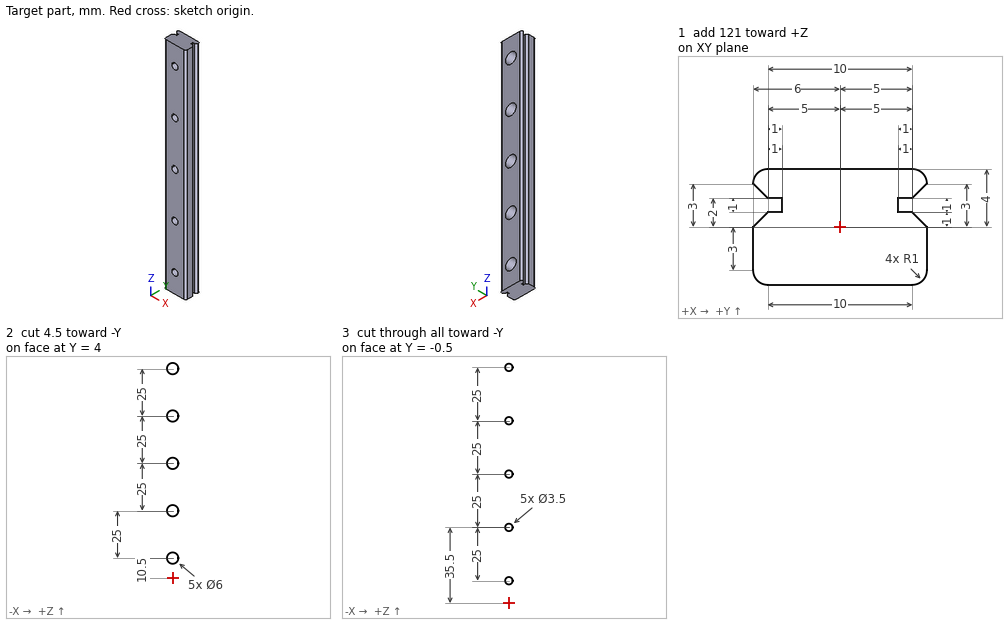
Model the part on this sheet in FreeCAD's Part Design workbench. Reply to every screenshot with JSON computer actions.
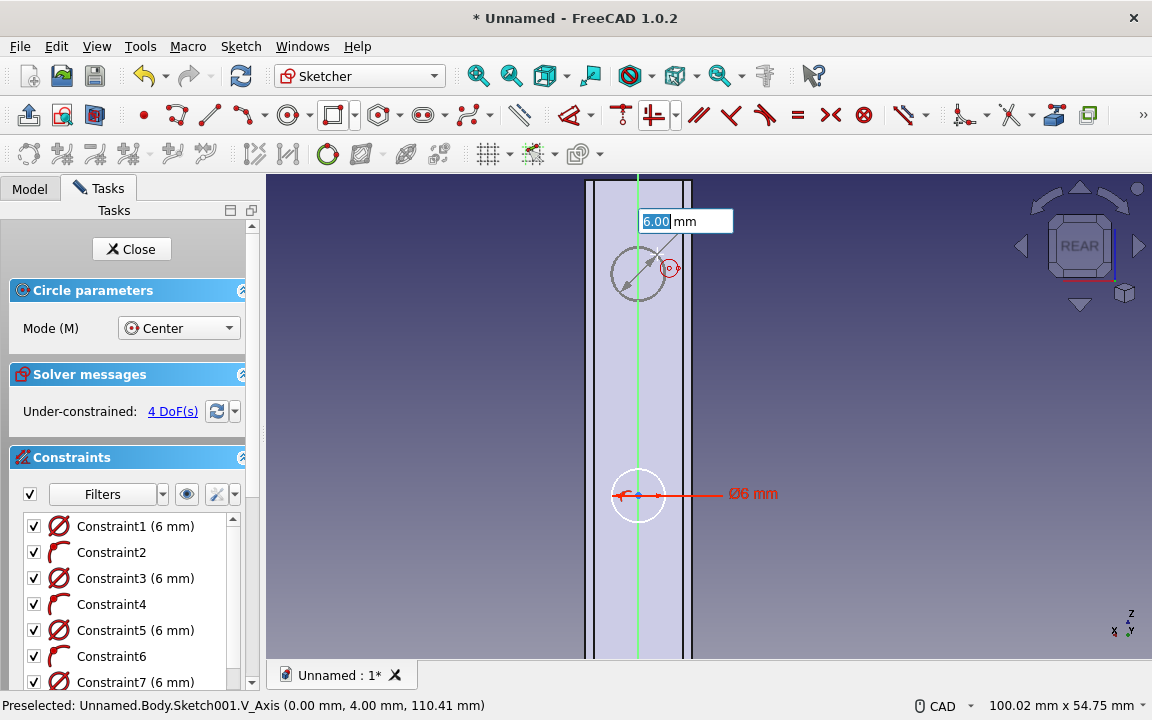
{"action": "type", "text": "6"}
{"action": "key", "text": "Return"}
{"action": "key", "text": "Escape"}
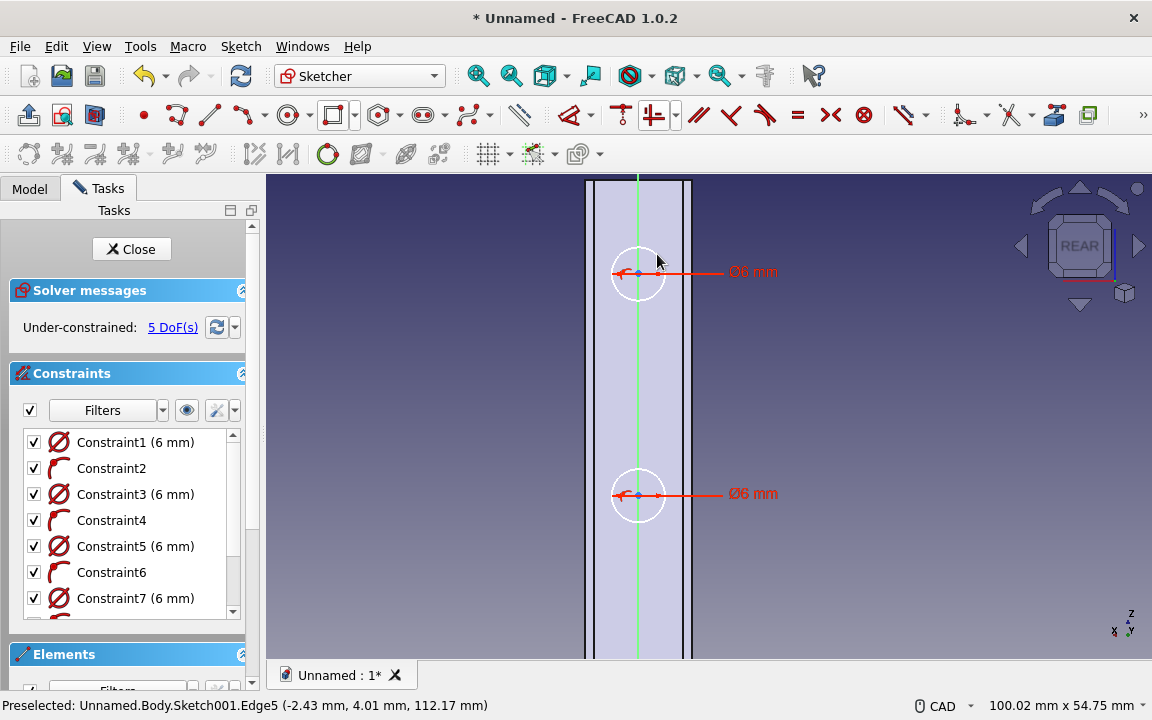
{"action": "left_click", "coordinate": [568, 116]}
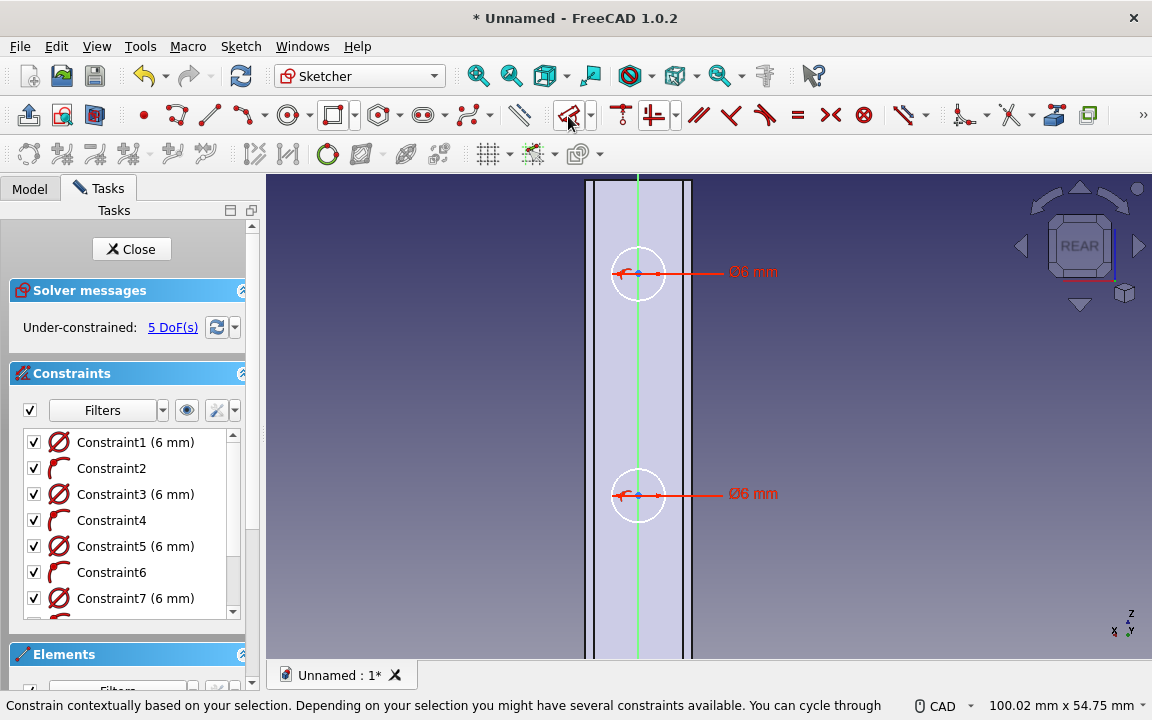
{"action": "scroll", "coordinate": [641, 273], "scroll_direction": "down", "scroll_amount": 6}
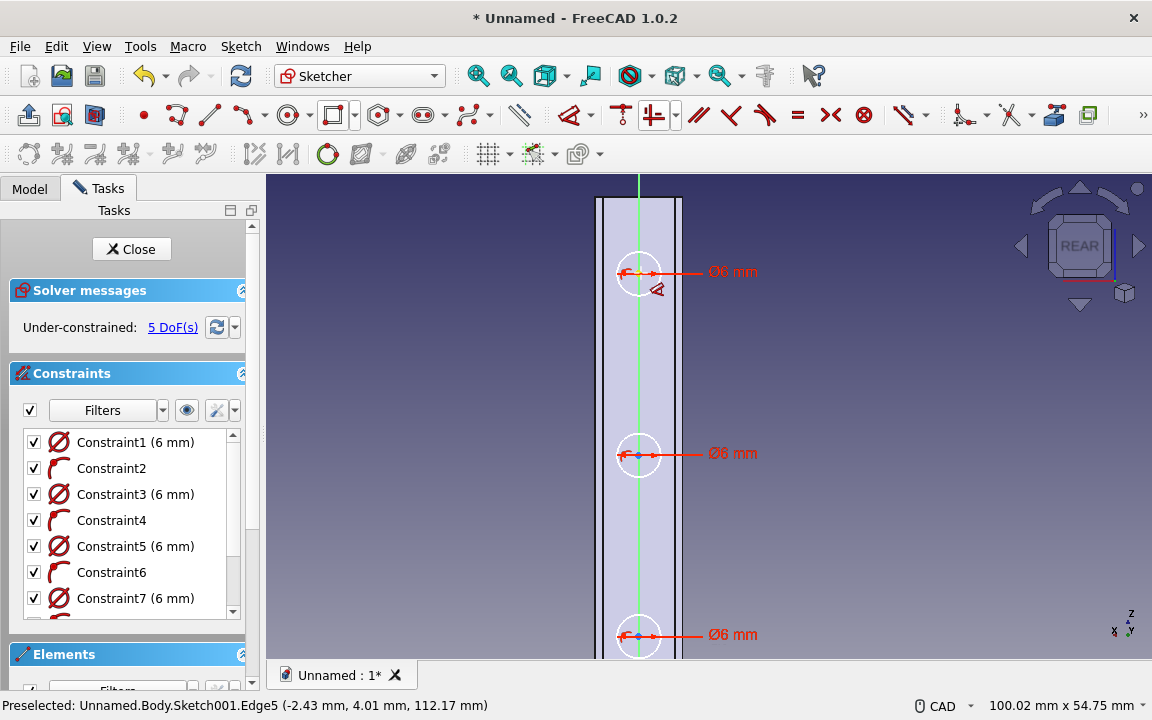
{"action": "left_click", "coordinate": [641, 540]}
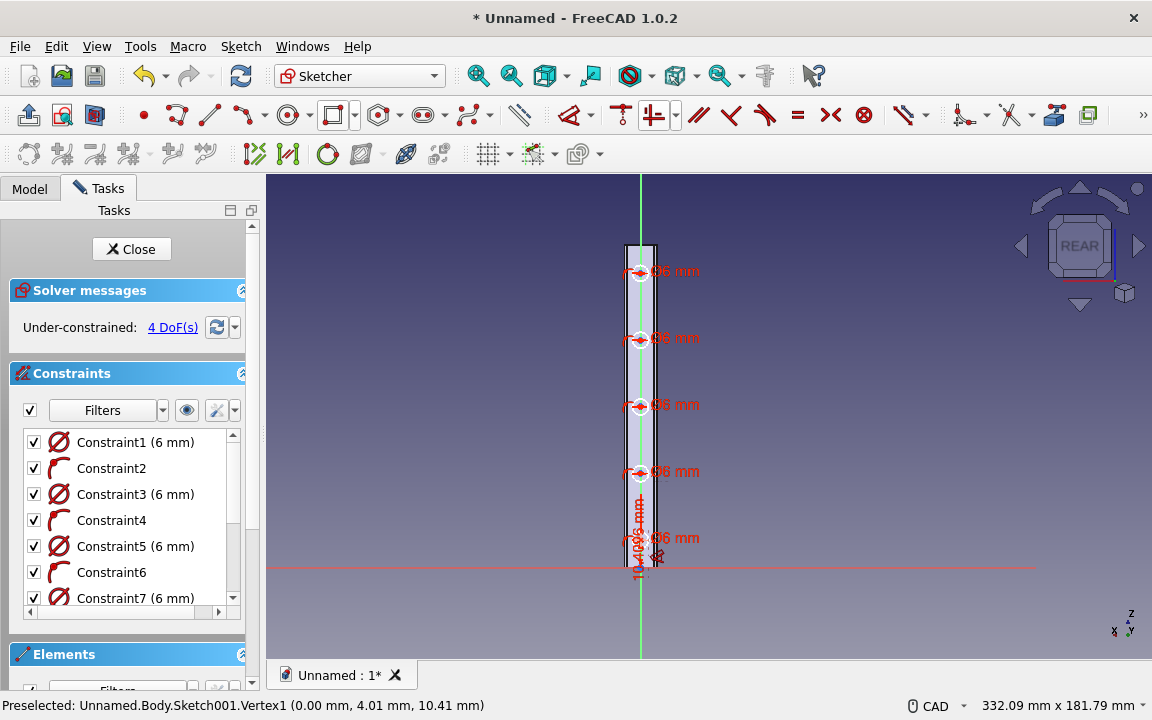
{"action": "left_click", "coordinate": [641, 474]}
{"action": "left_click", "coordinate": [675, 507]}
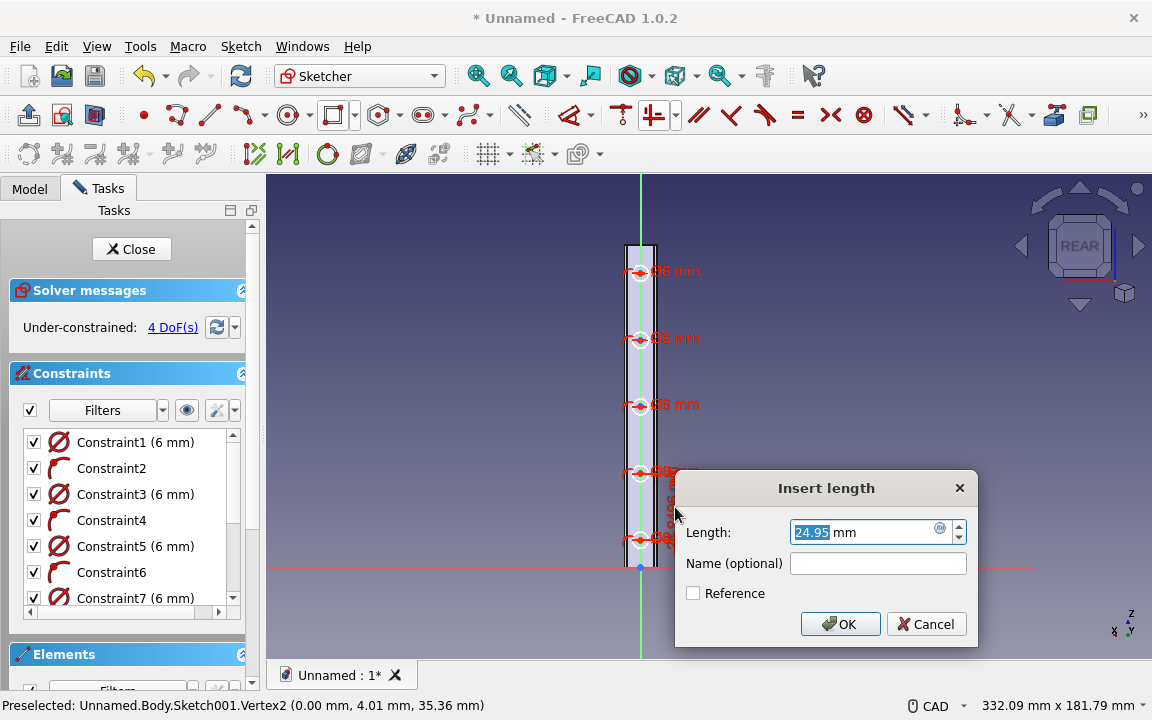
{"action": "type", "text": "25"}
{"action": "key", "text": "Return"}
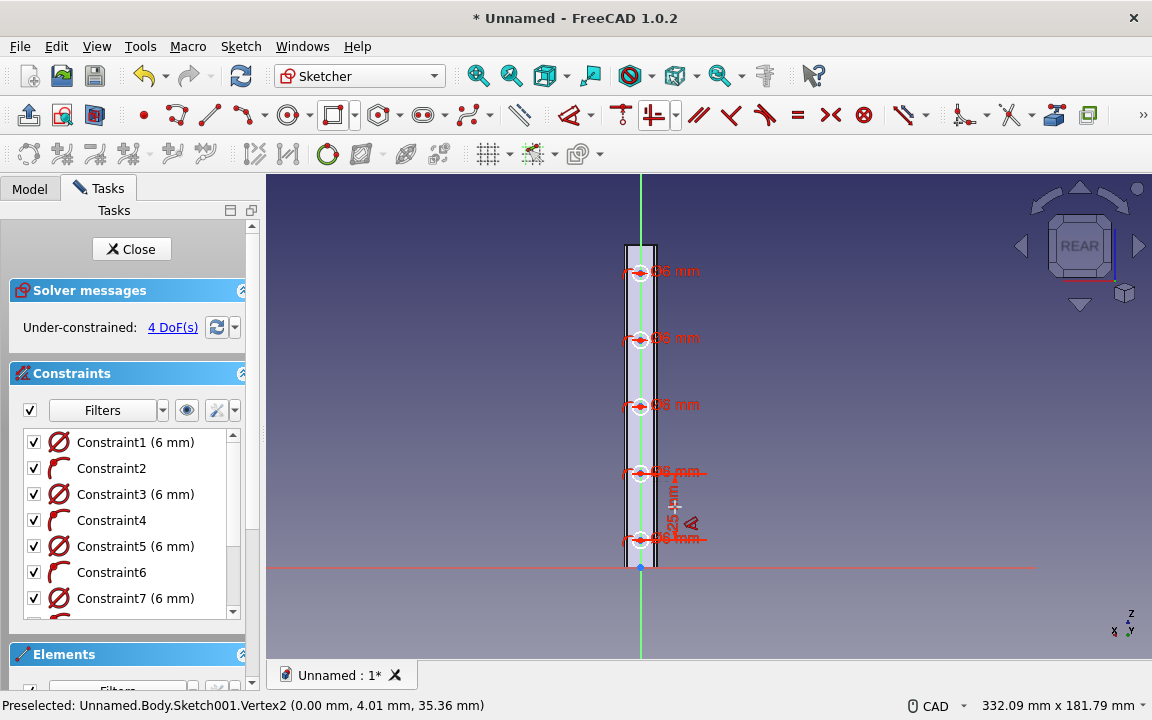
{"action": "left_click", "coordinate": [641, 474]}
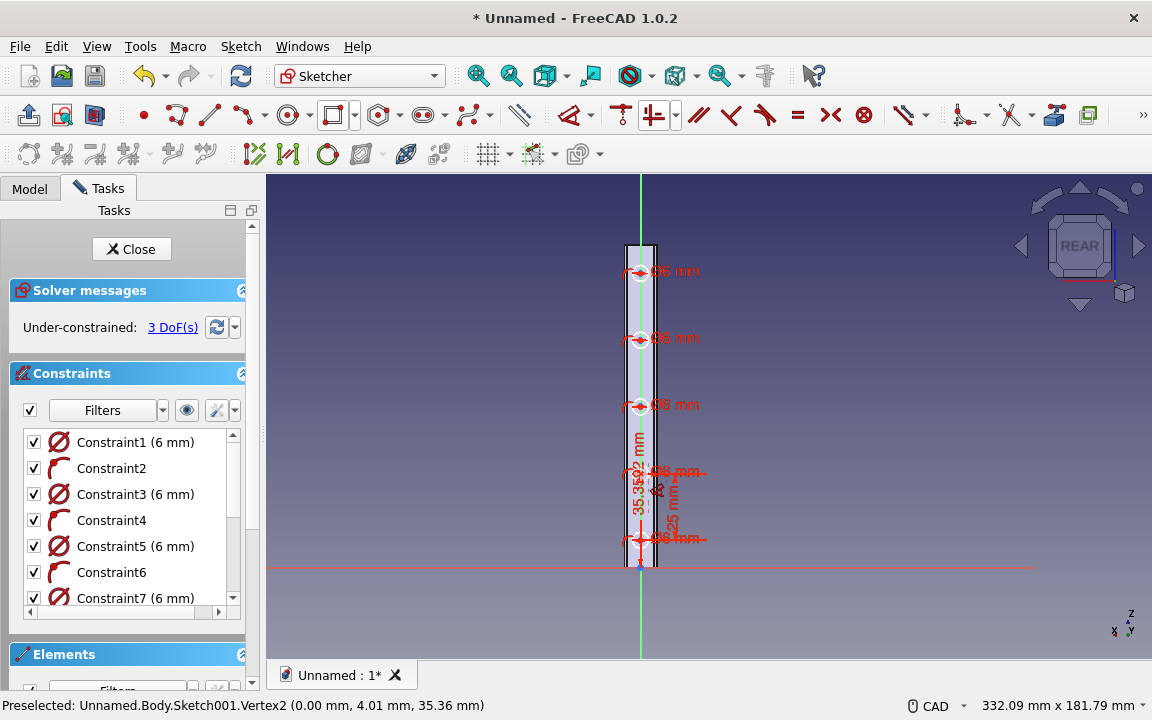
{"action": "left_click", "coordinate": [641, 407]}
{"action": "left_click", "coordinate": [675, 440]}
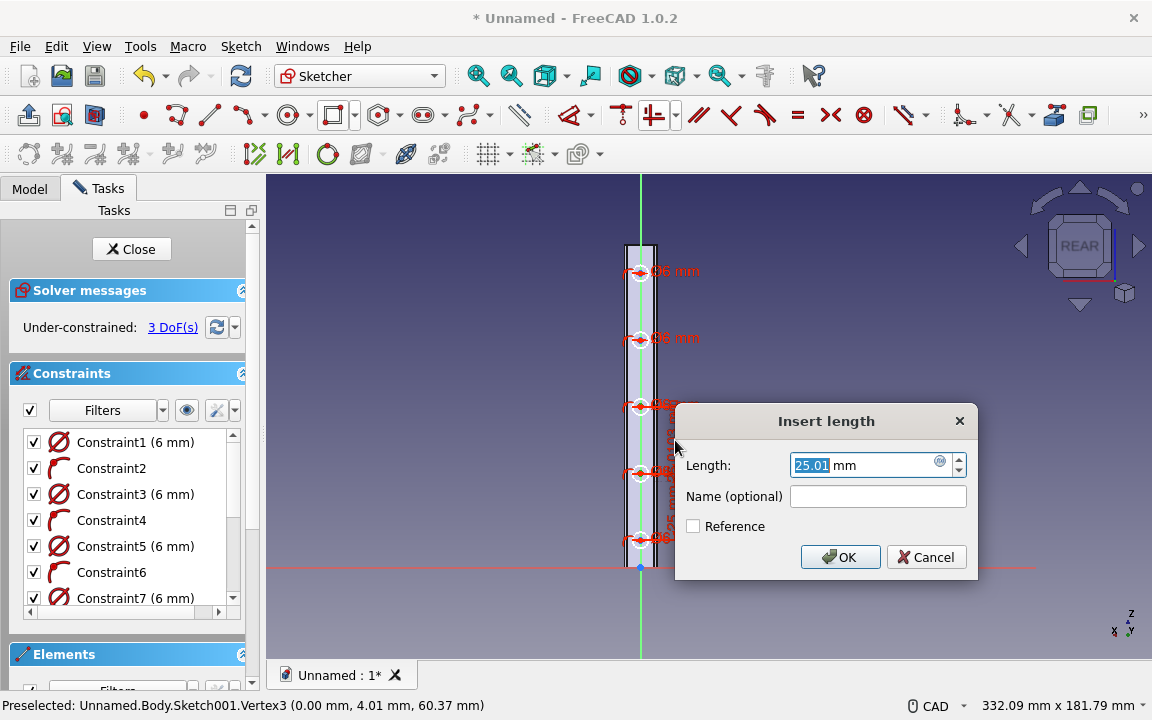
{"action": "type", "text": "25"}
{"action": "key", "text": "Return"}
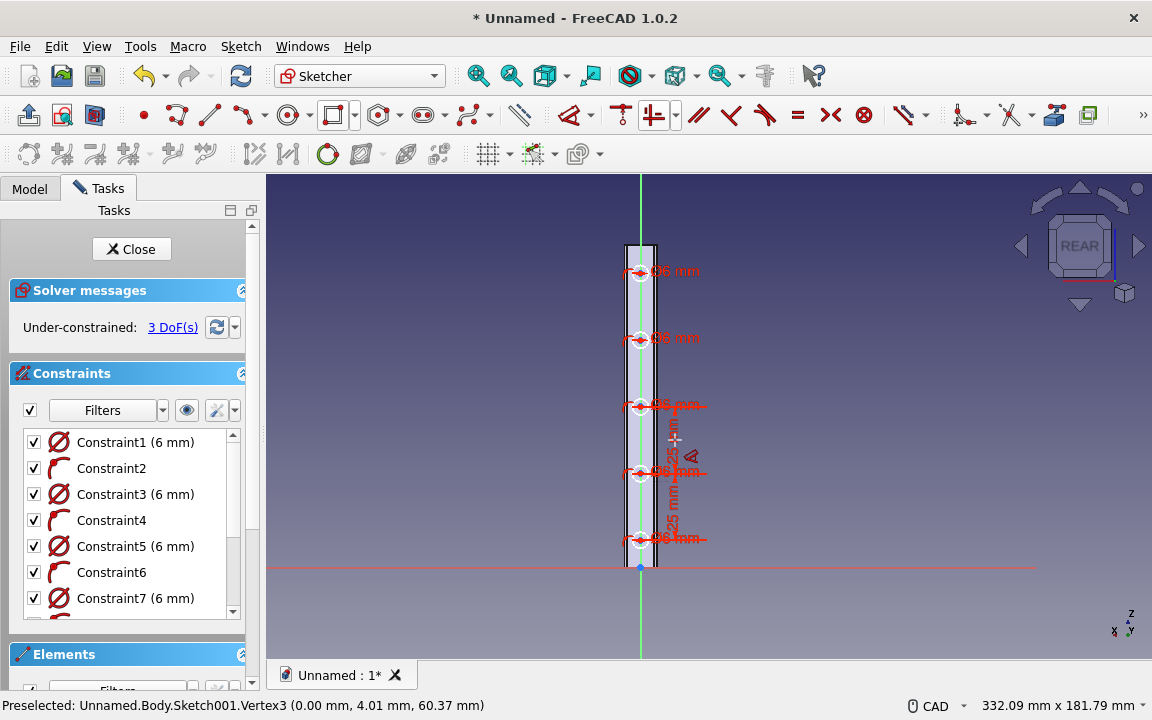
{"action": "left_click", "coordinate": [641, 407]}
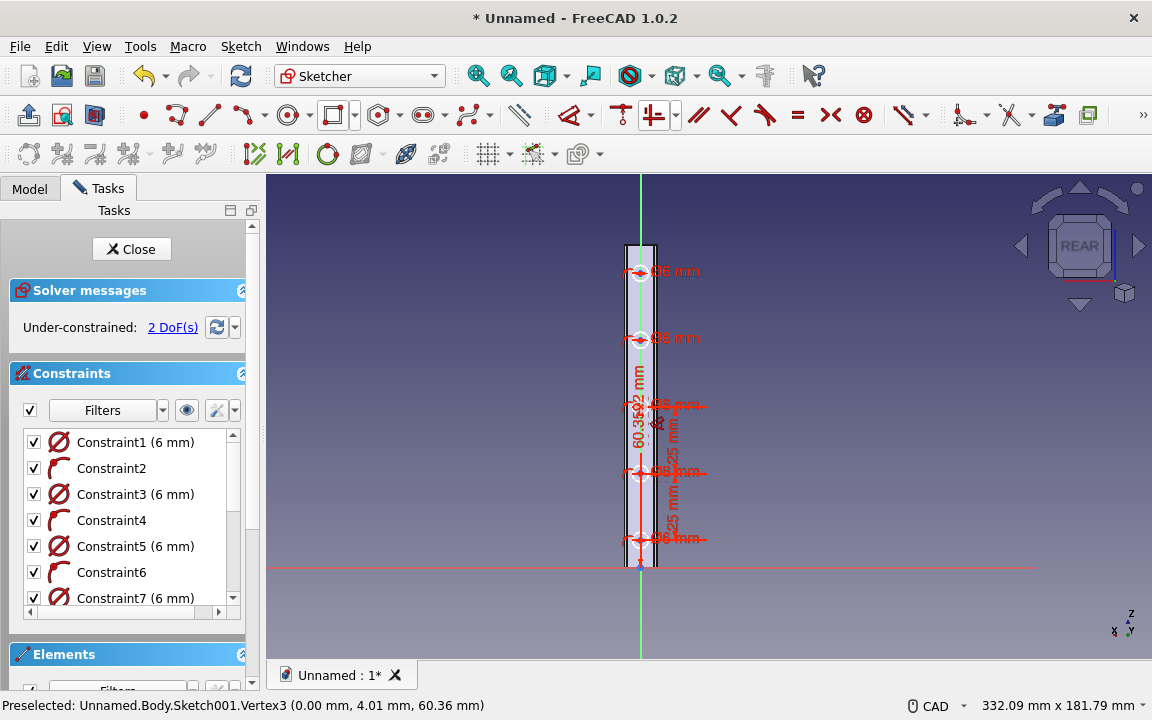
{"action": "left_click", "coordinate": [641, 340]}
{"action": "left_click", "coordinate": [675, 374]}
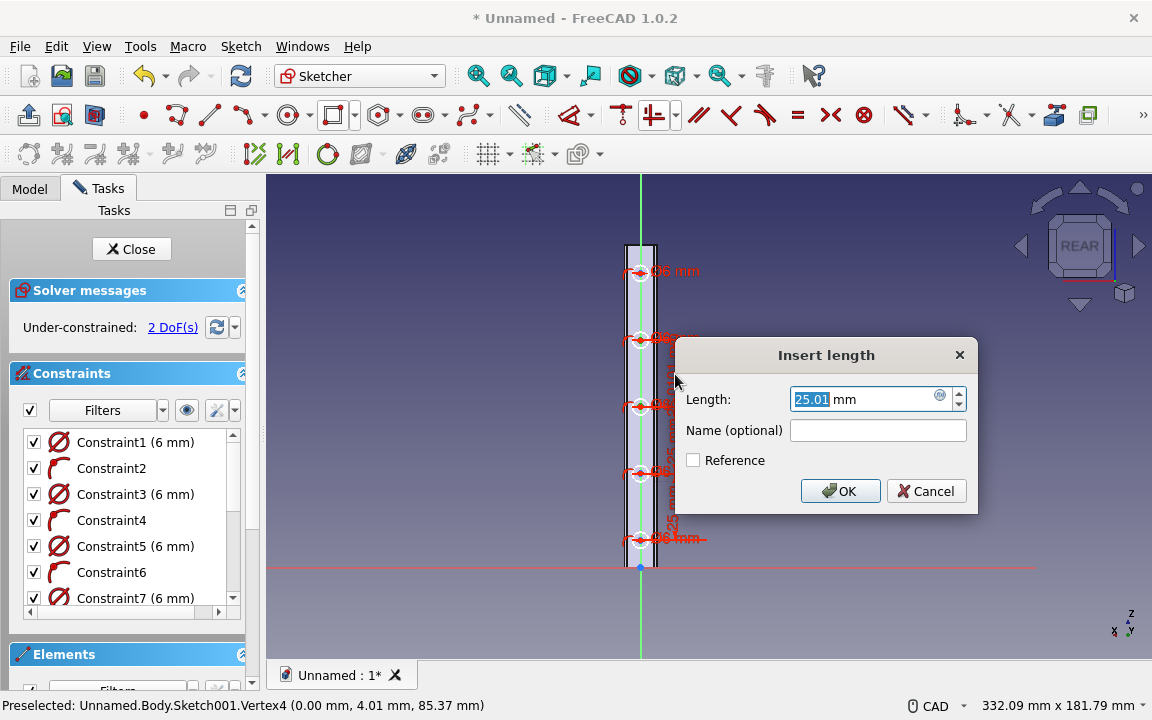
{"action": "type", "text": "25"}
{"action": "key", "text": "Return"}